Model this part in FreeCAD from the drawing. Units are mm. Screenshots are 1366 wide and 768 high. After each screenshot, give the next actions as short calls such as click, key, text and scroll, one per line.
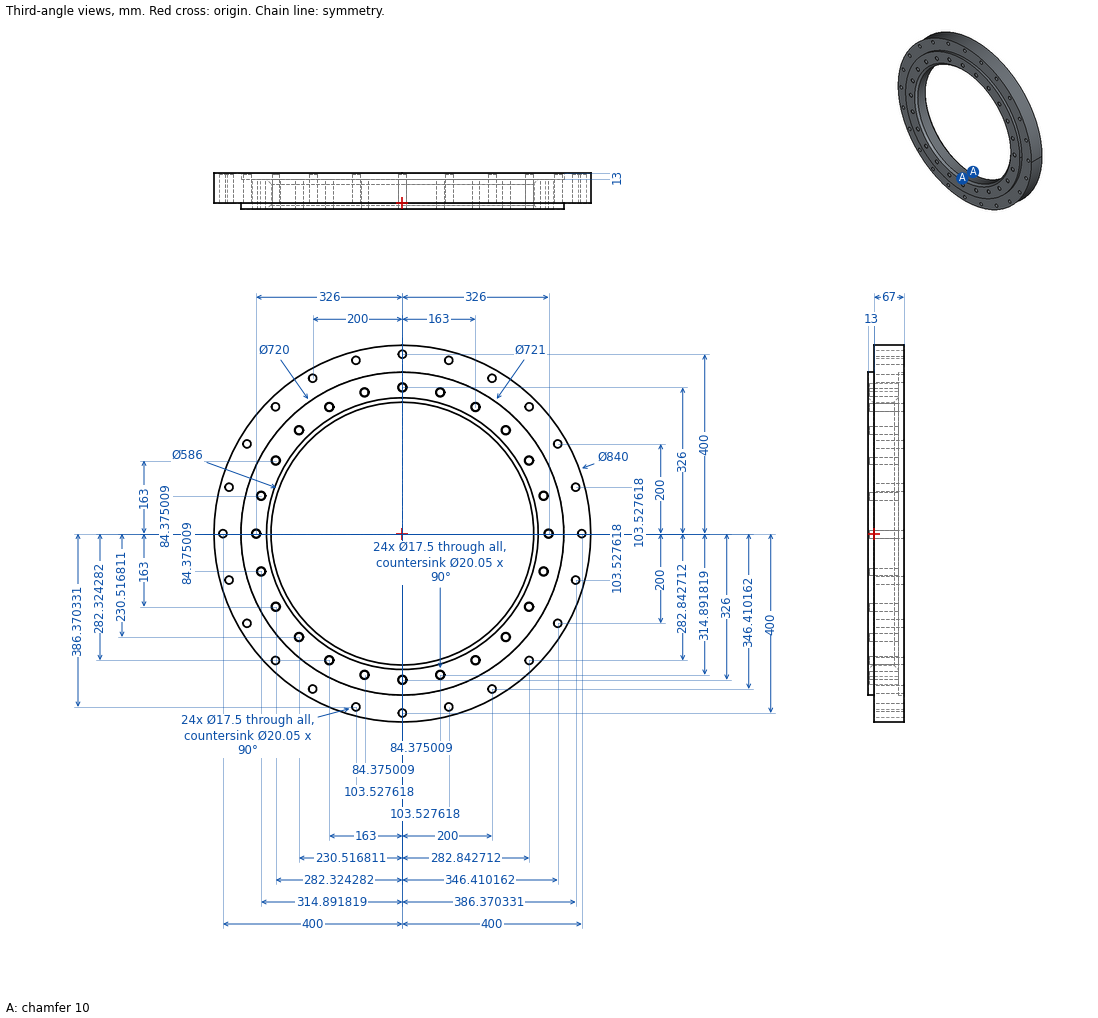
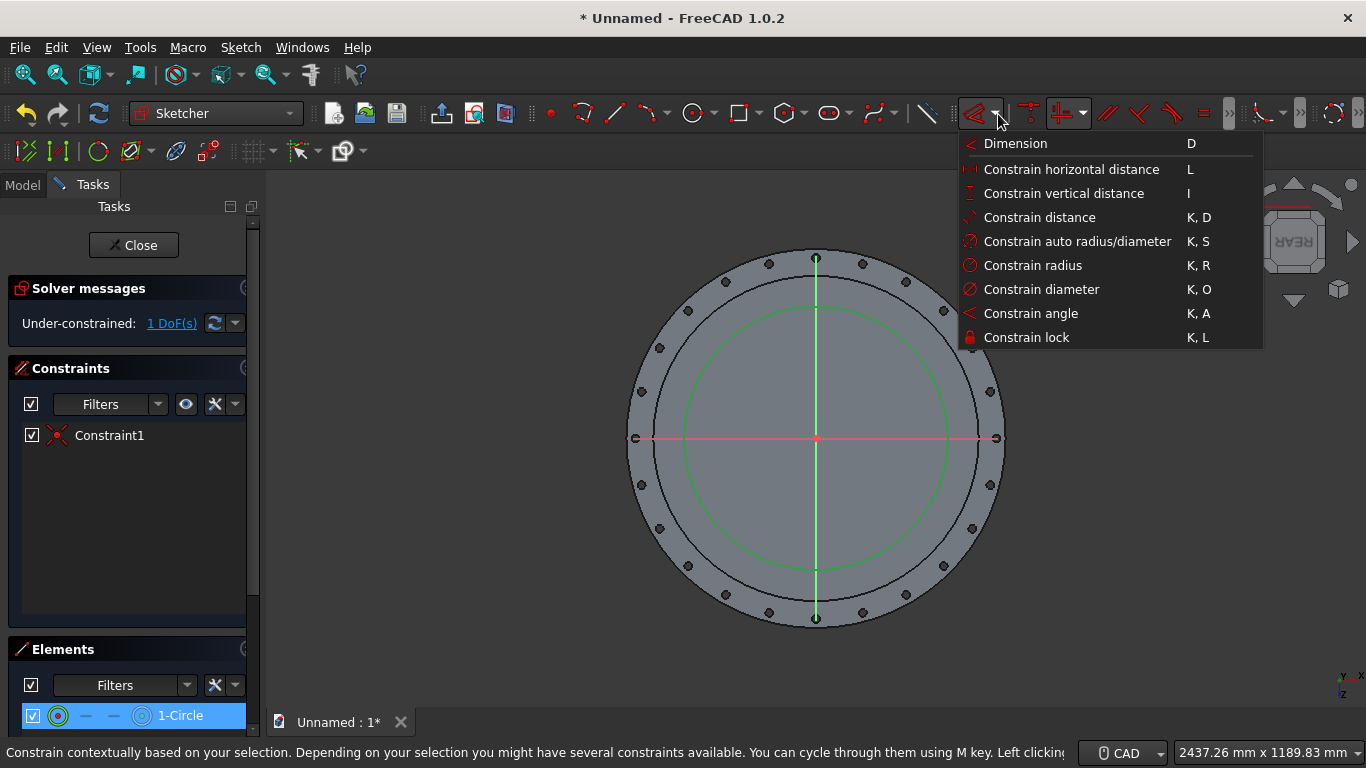
click(1111, 289)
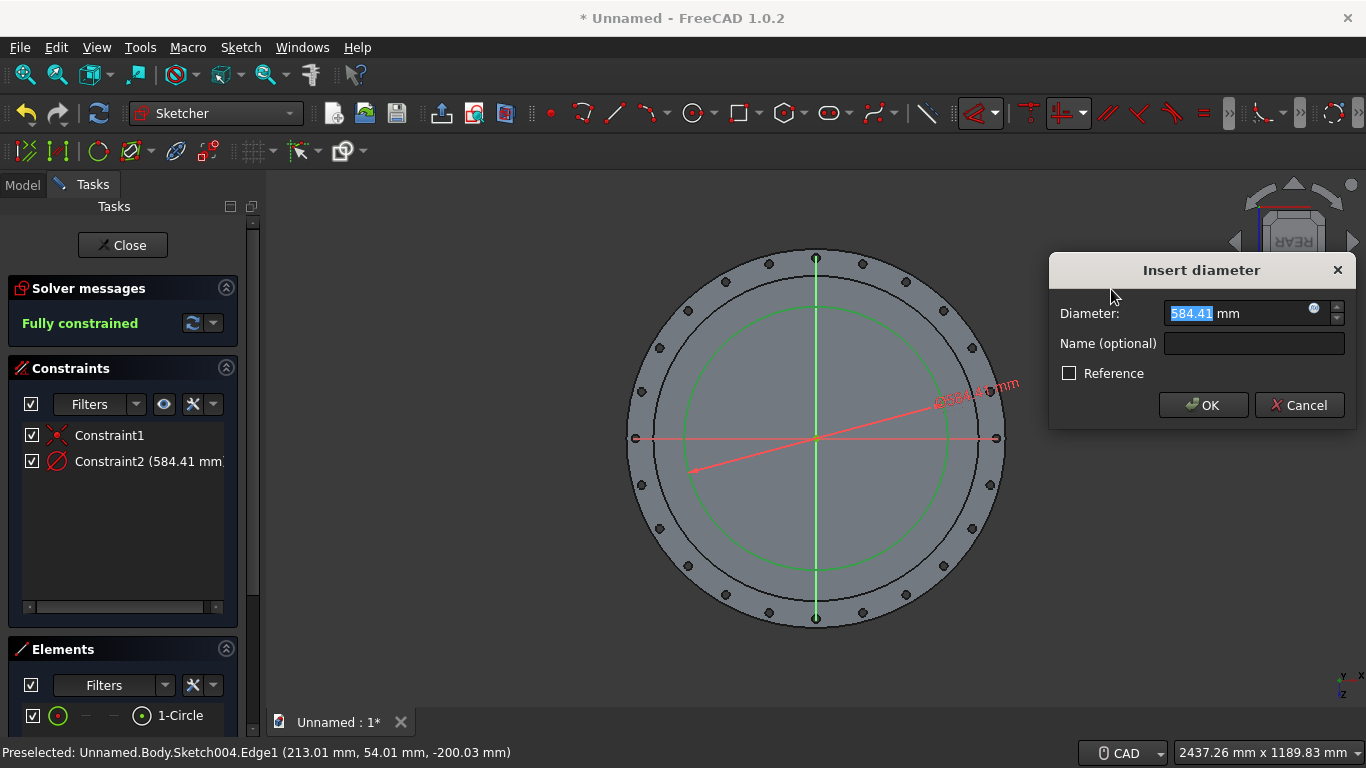
text(586)
key(Return)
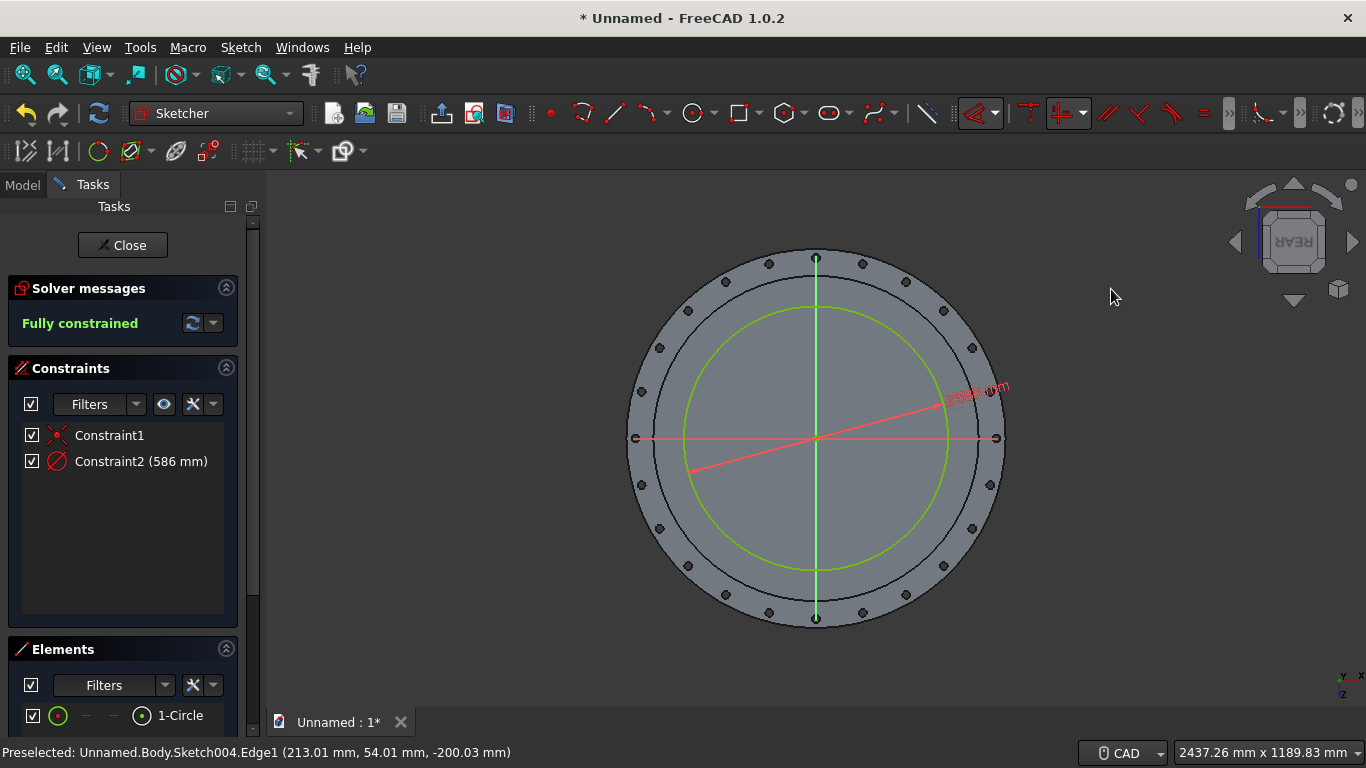
click(123, 245)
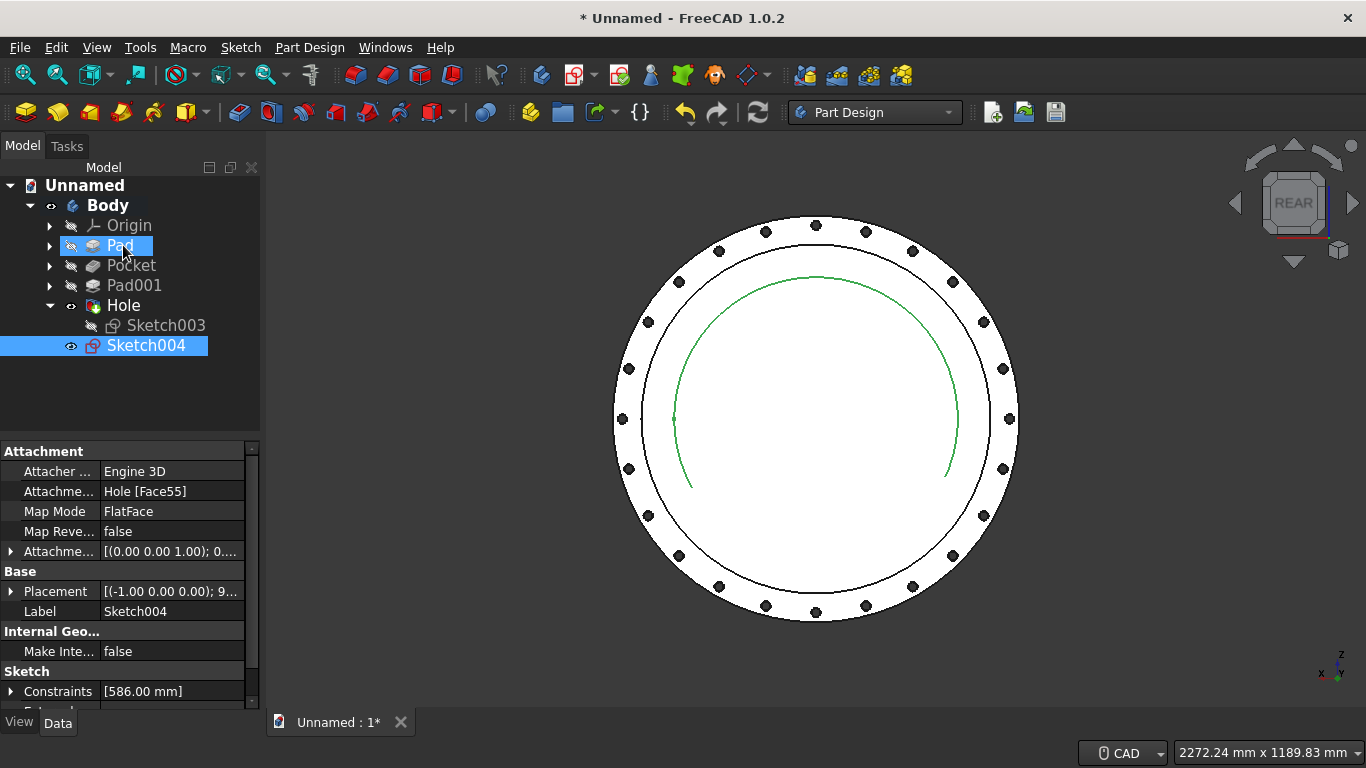
click(240, 112)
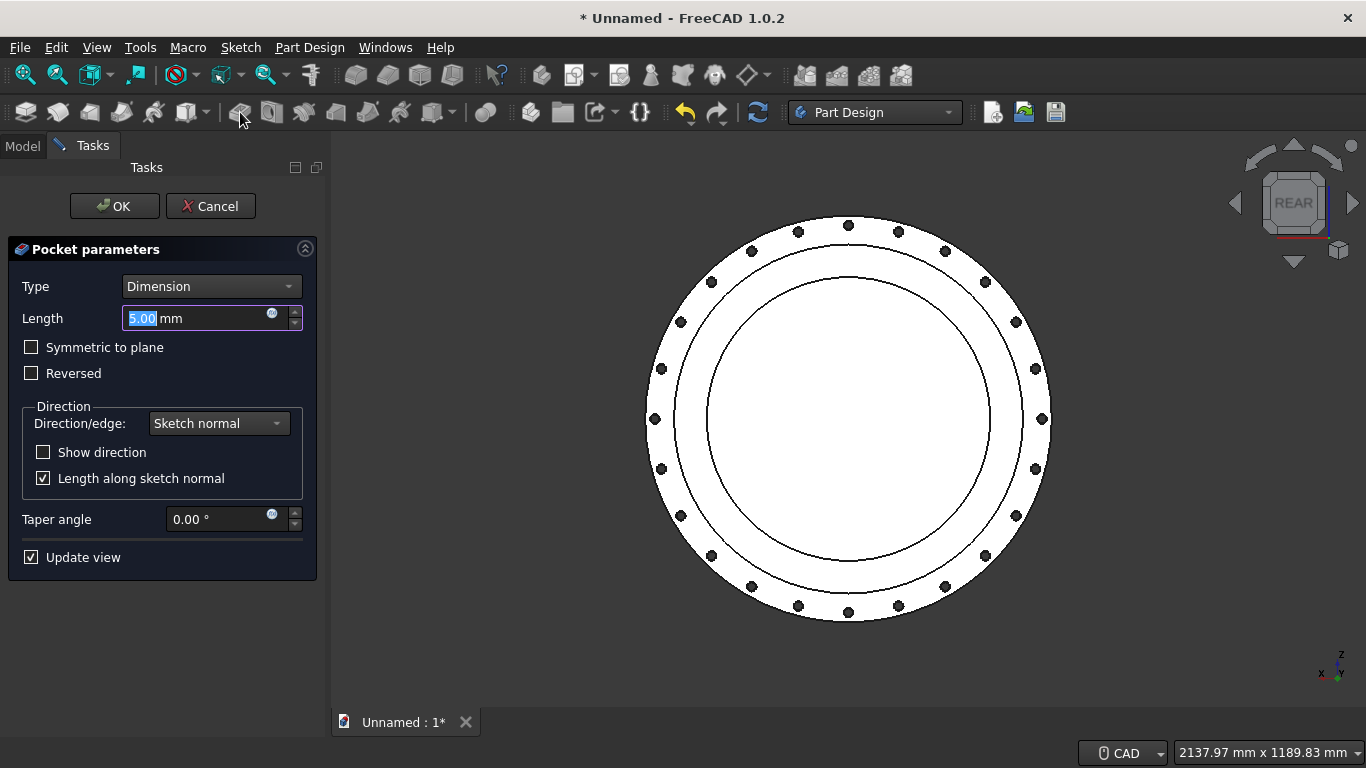
click(212, 286)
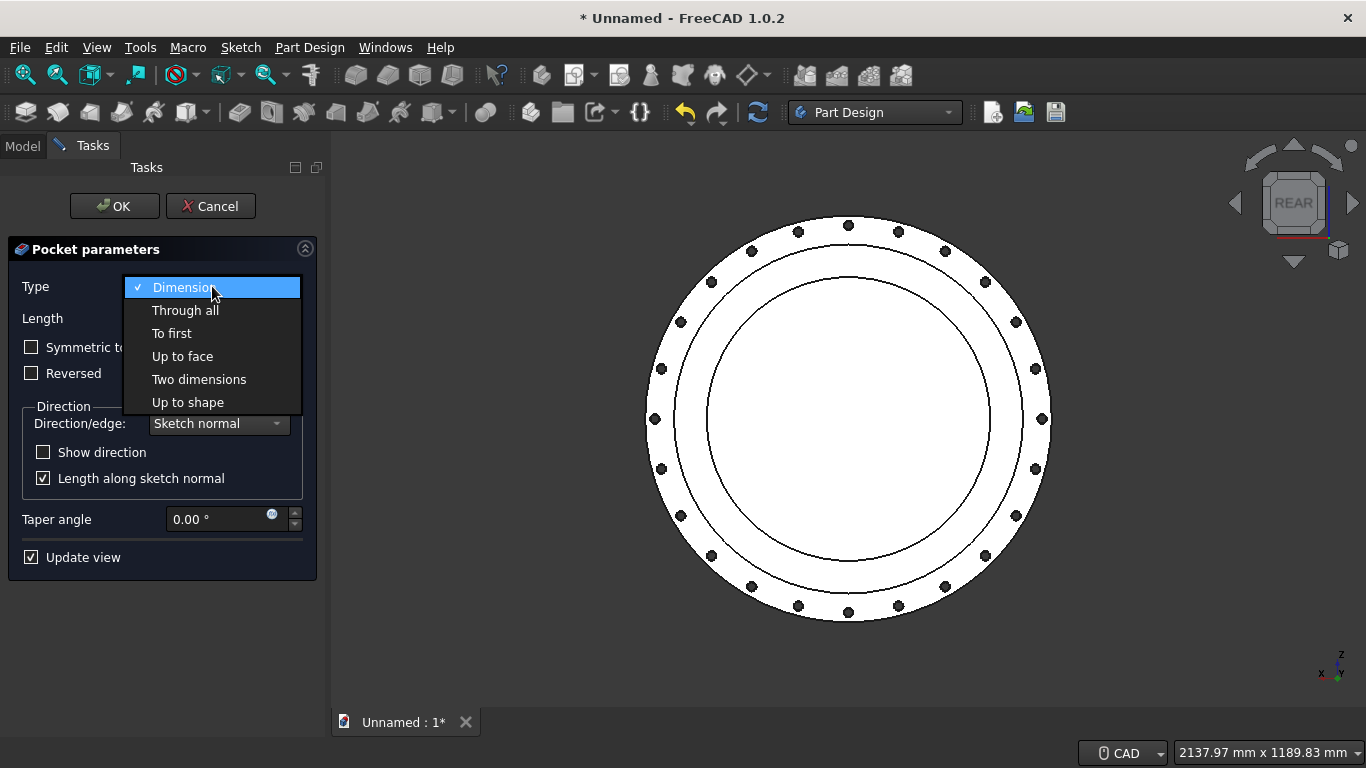
click(212, 310)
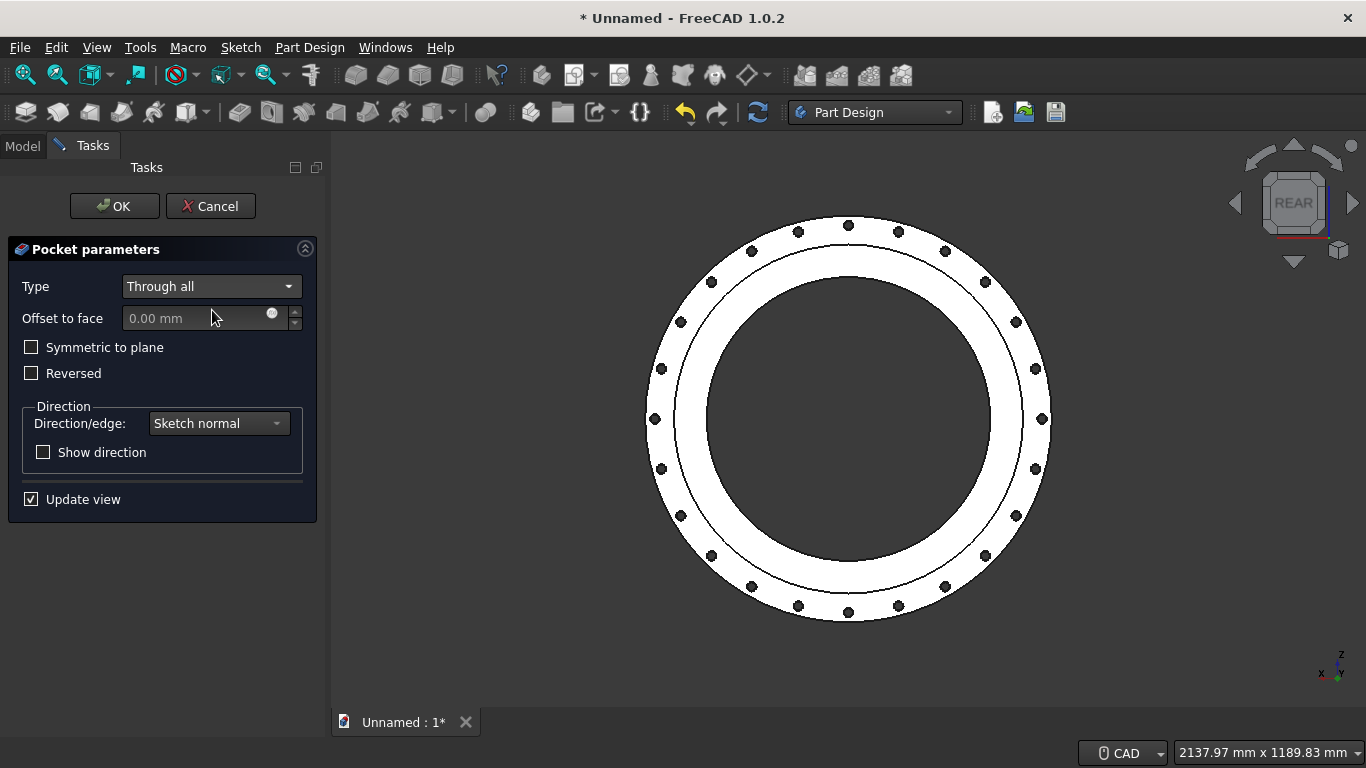
click(115, 206)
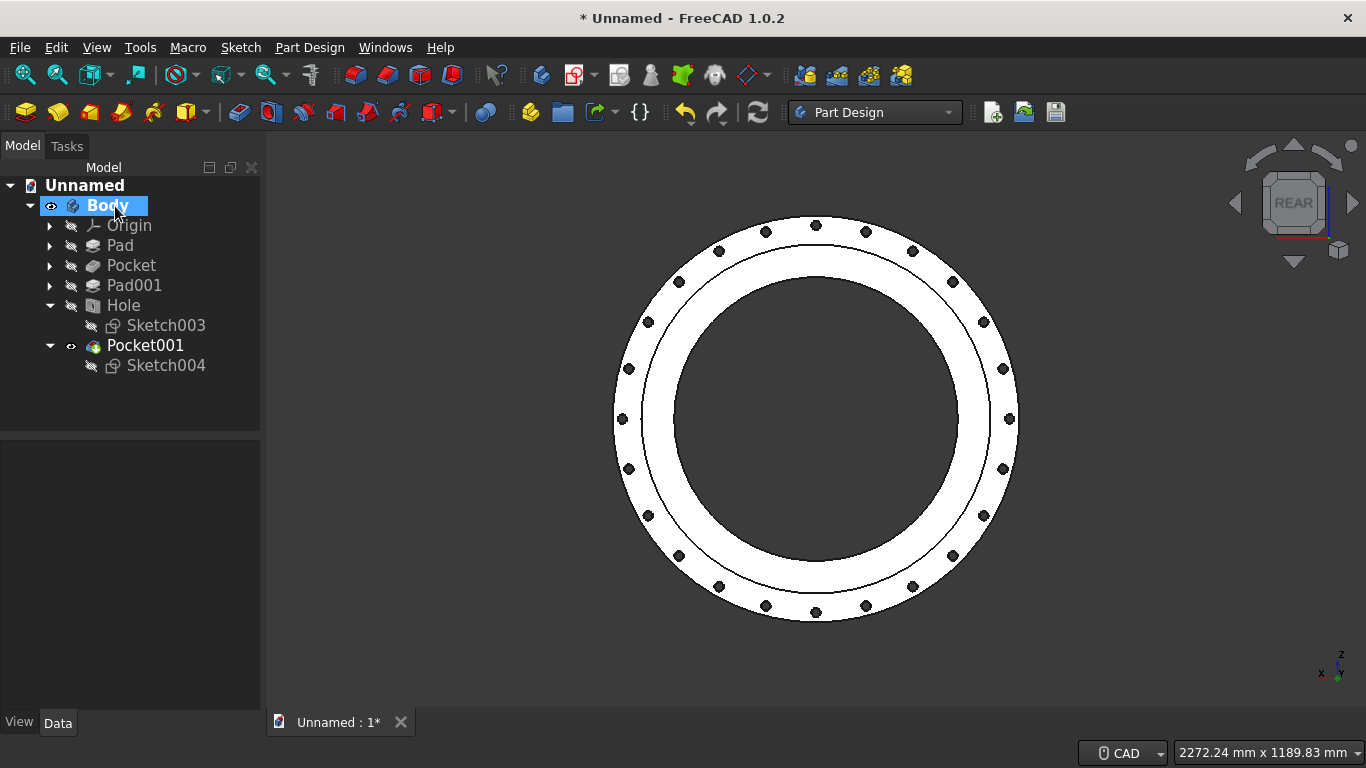
click(931, 335)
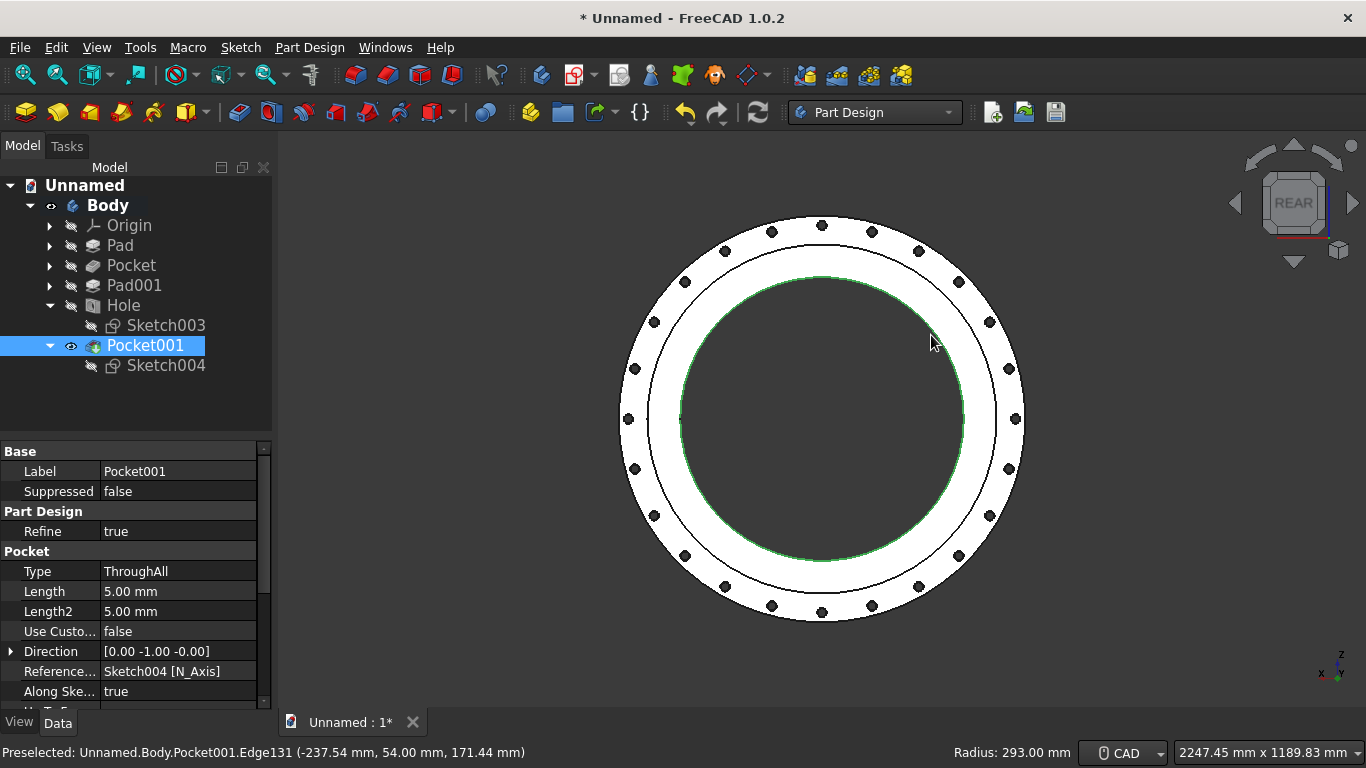
key(0)